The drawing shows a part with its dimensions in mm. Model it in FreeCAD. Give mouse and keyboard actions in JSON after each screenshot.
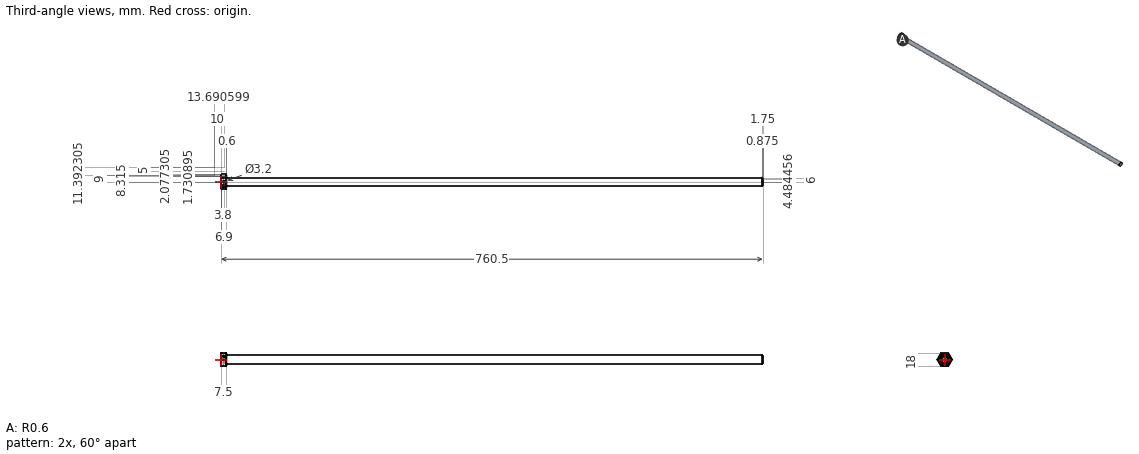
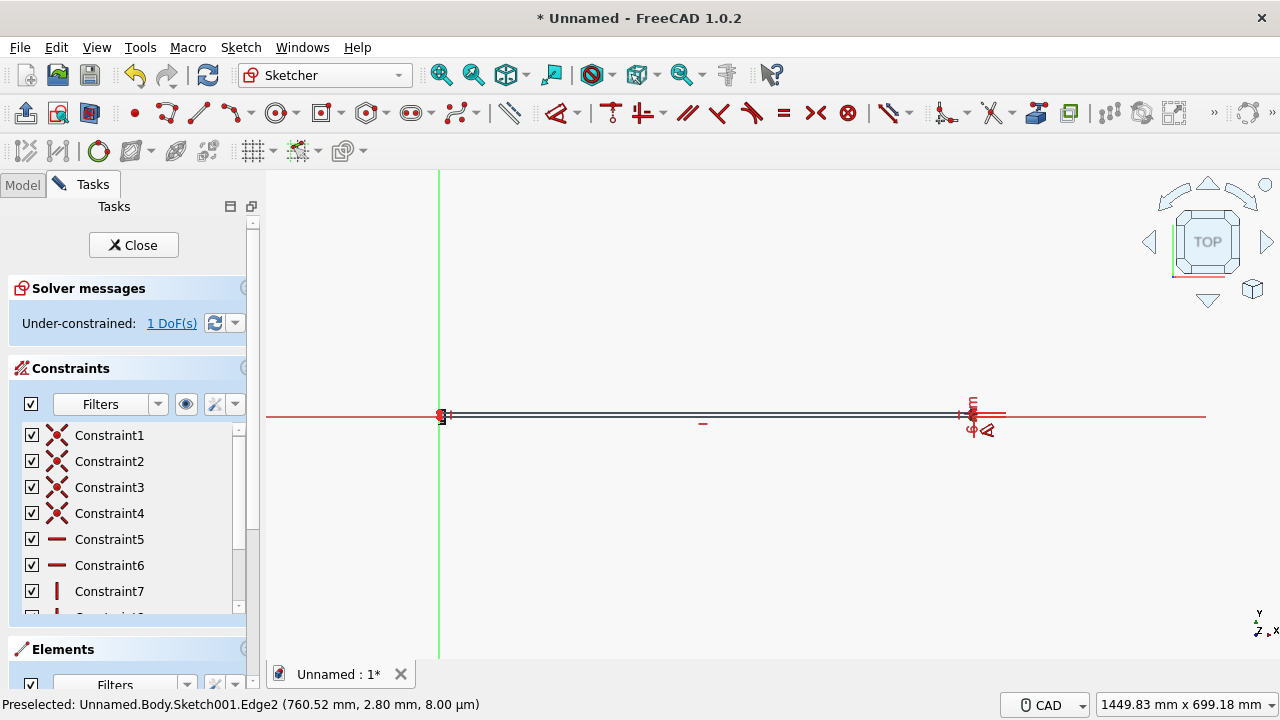
{"action": "scroll", "coordinate": [599, 417], "scroll_direction": "up", "scroll_amount": 6}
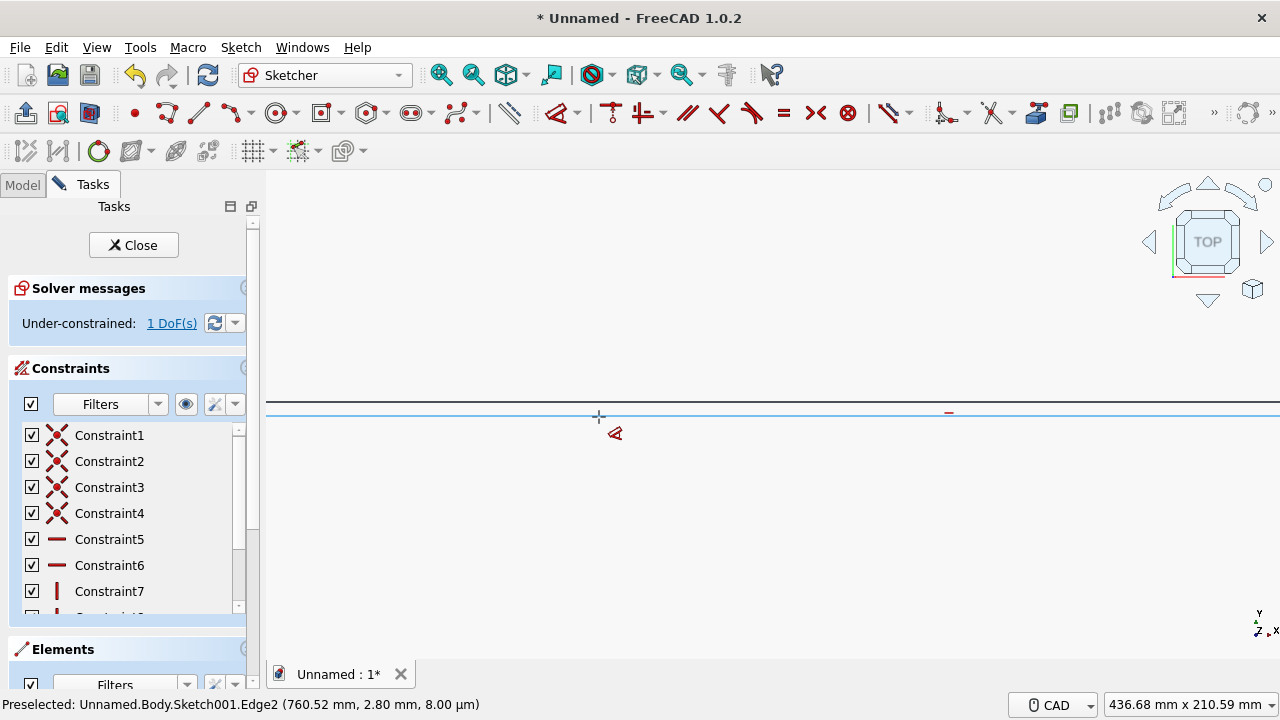
{"action": "left_click", "coordinate": [598, 416]}
{"action": "left_click", "coordinate": [704, 450]}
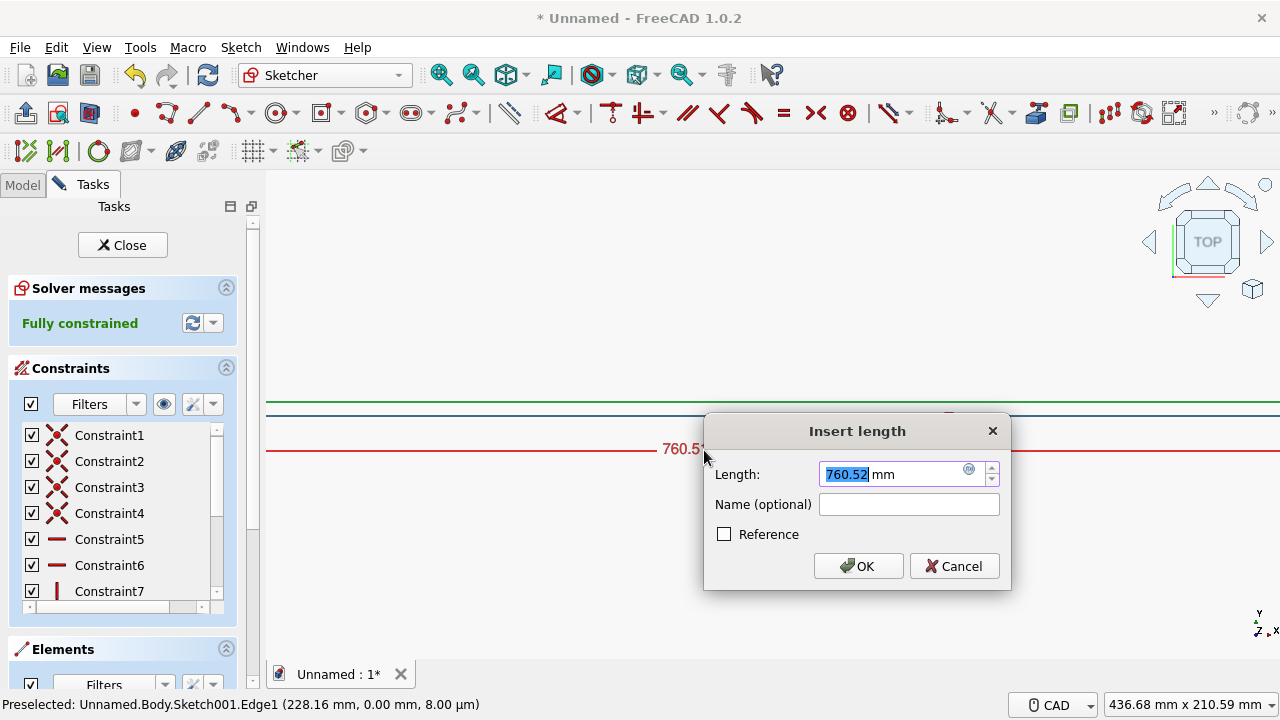
{"action": "type", "text": "760.5"}
{"action": "key", "text": "Return"}
{"action": "key", "text": "Escape"}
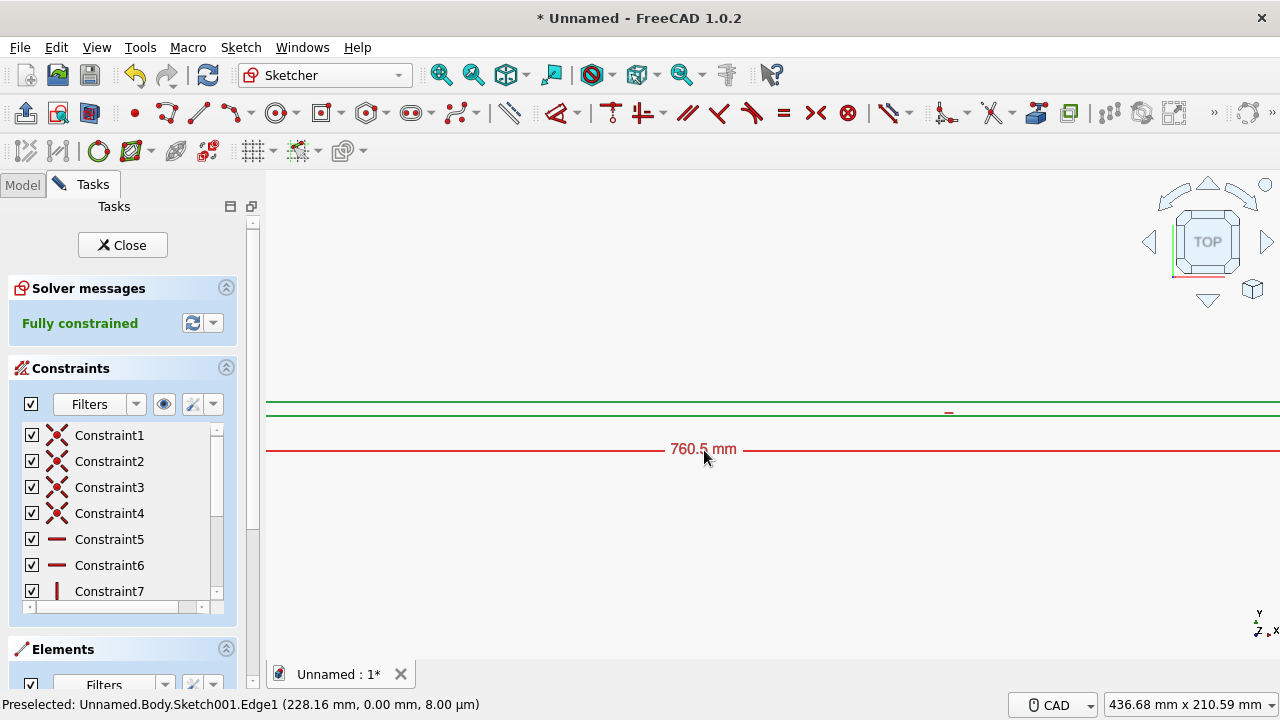
{"action": "left_click", "coordinate": [123, 245]}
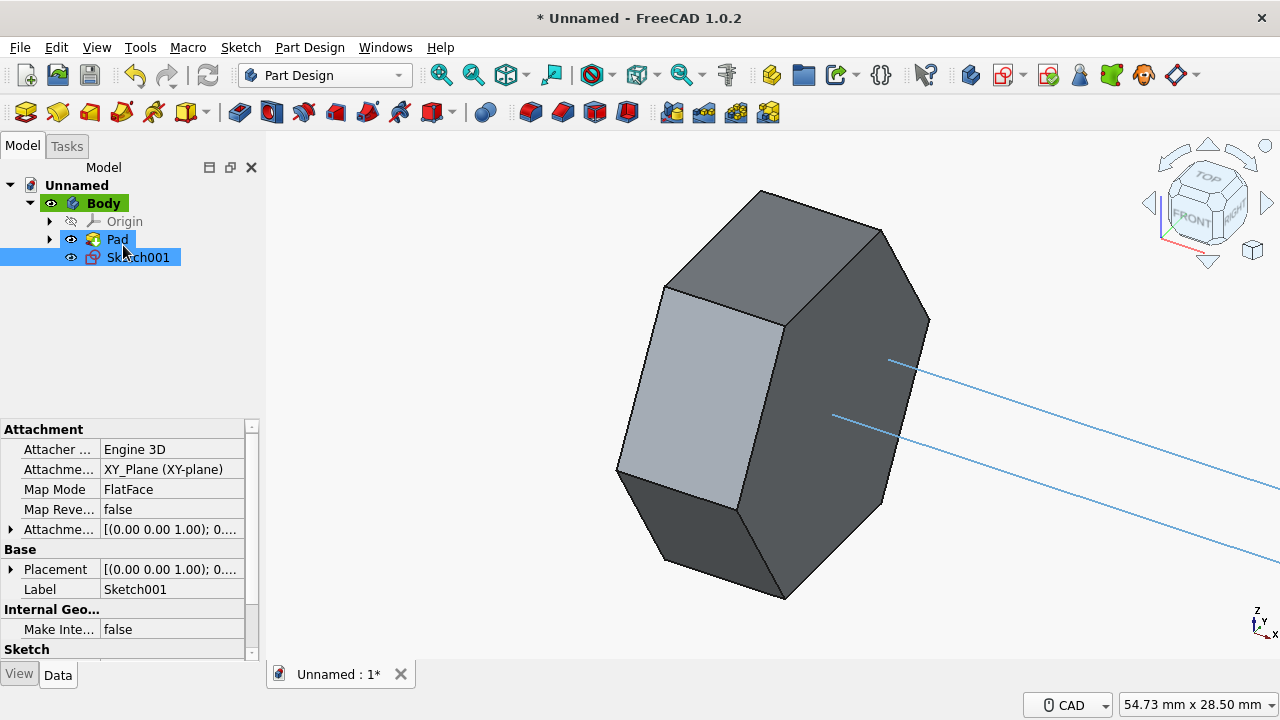
{"action": "left_click", "coordinate": [58, 112]}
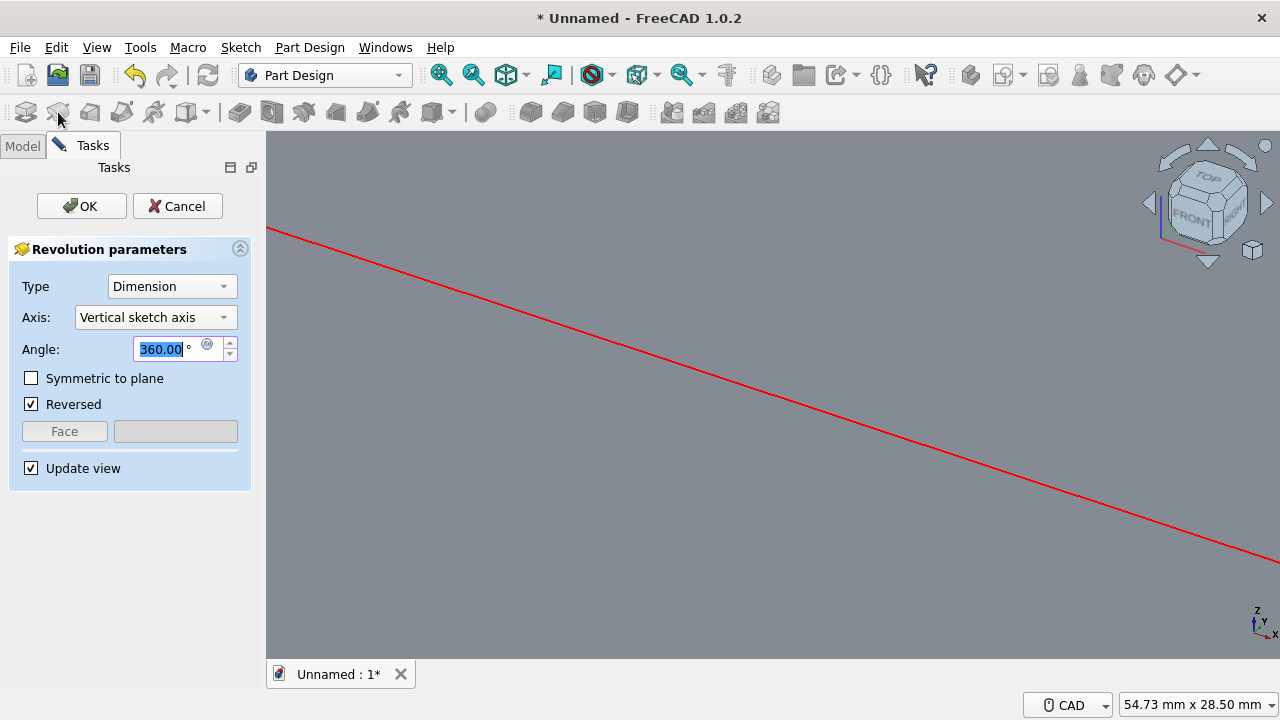
{"action": "left_click", "coordinate": [156, 318]}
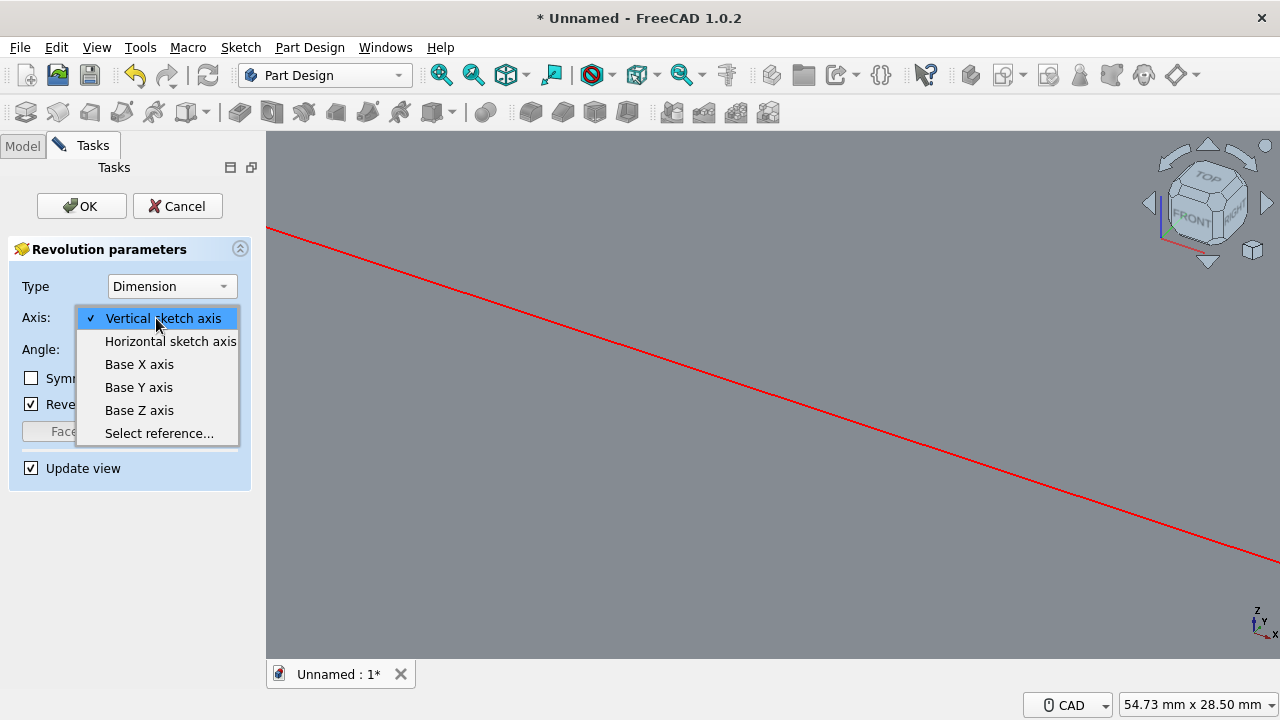
{"action": "left_click", "coordinate": [156, 342]}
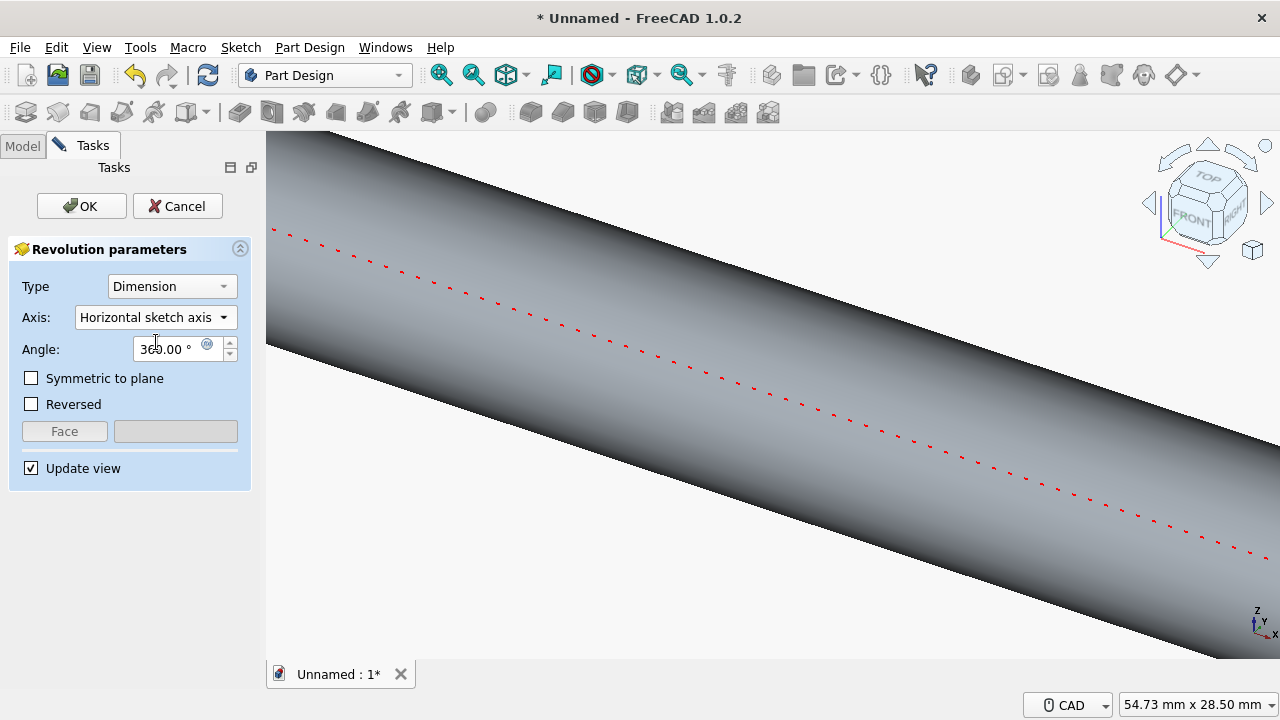
{"action": "left_click", "coordinate": [82, 206]}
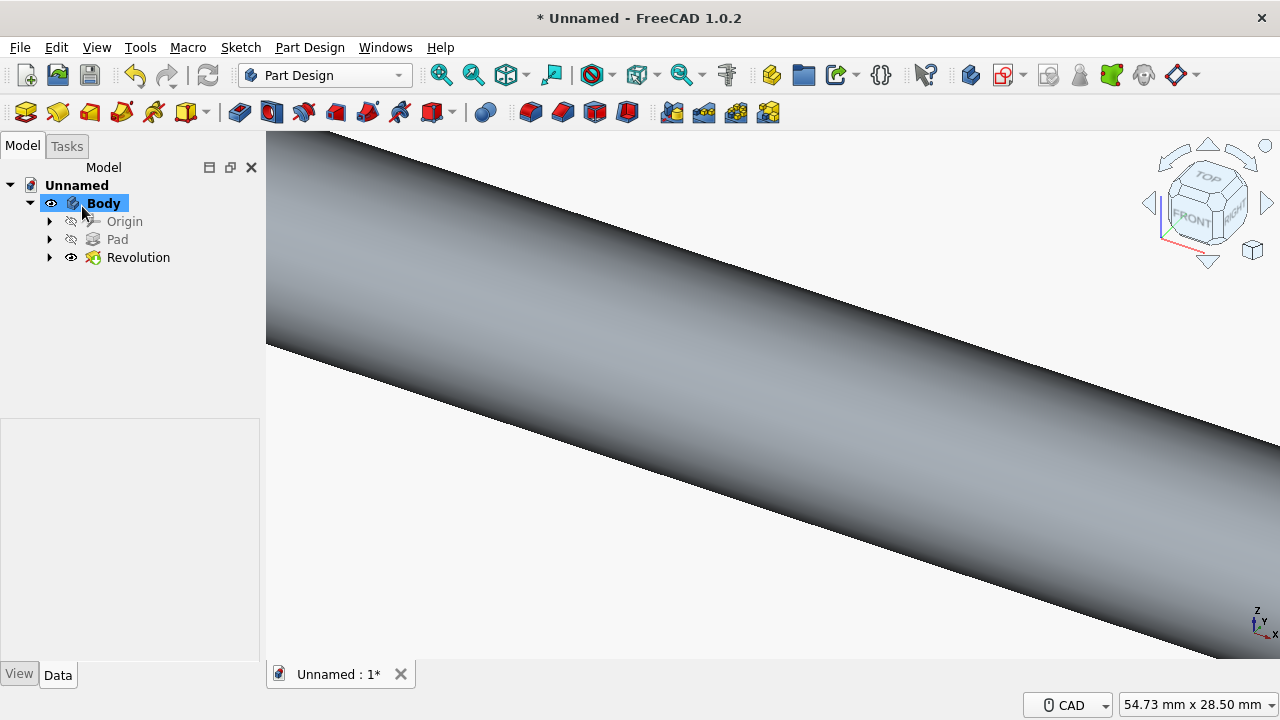
{"action": "left_click", "coordinate": [442, 76]}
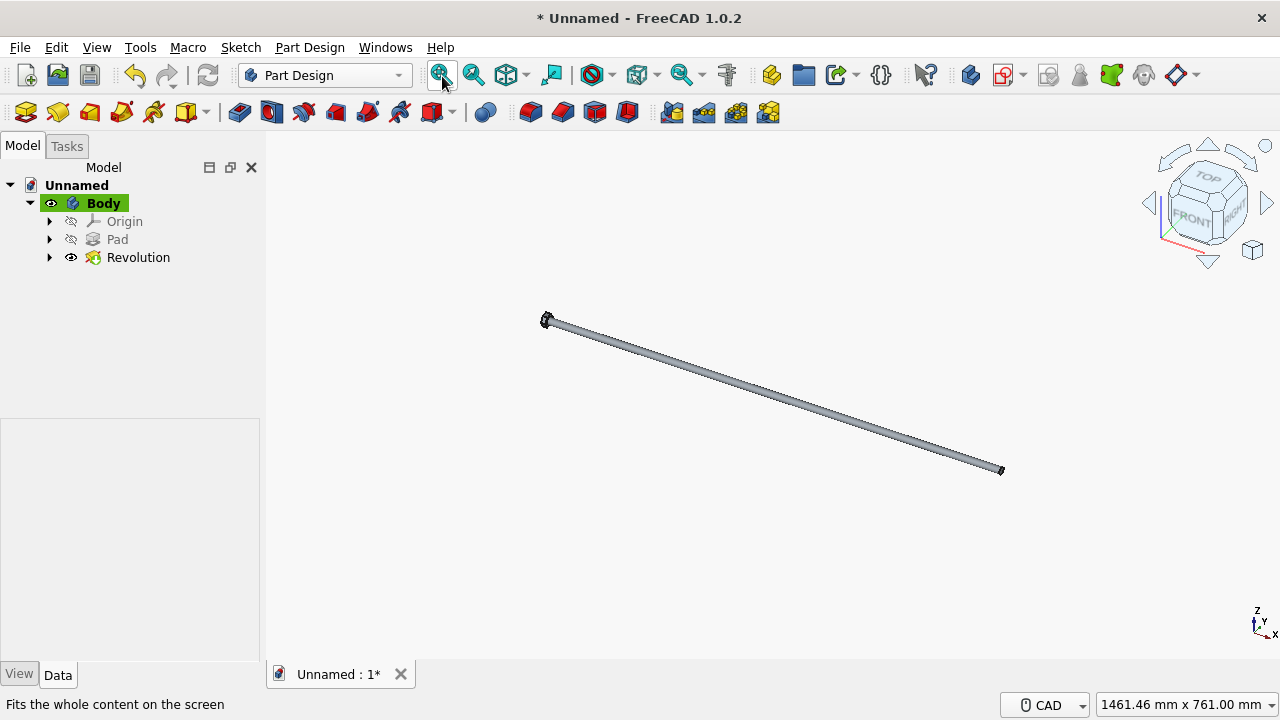
{"action": "left_click", "coordinate": [1004, 76]}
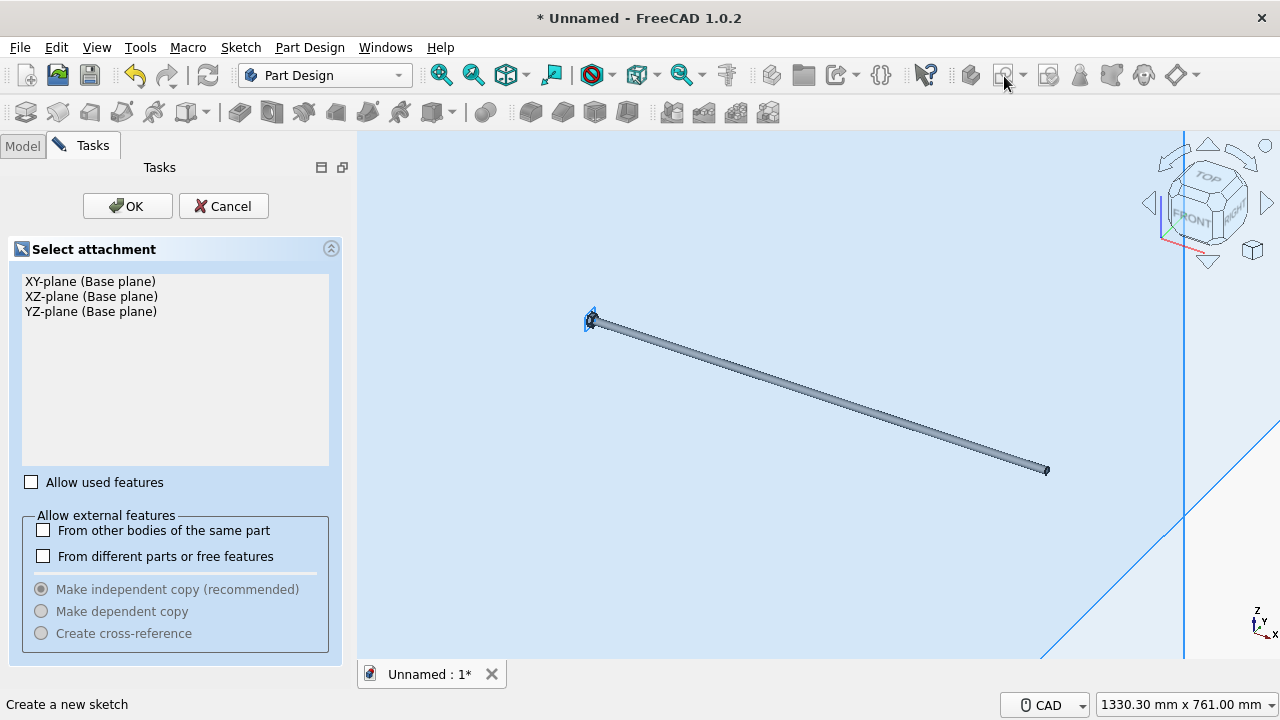
{"action": "left_click", "coordinate": [82, 282]}